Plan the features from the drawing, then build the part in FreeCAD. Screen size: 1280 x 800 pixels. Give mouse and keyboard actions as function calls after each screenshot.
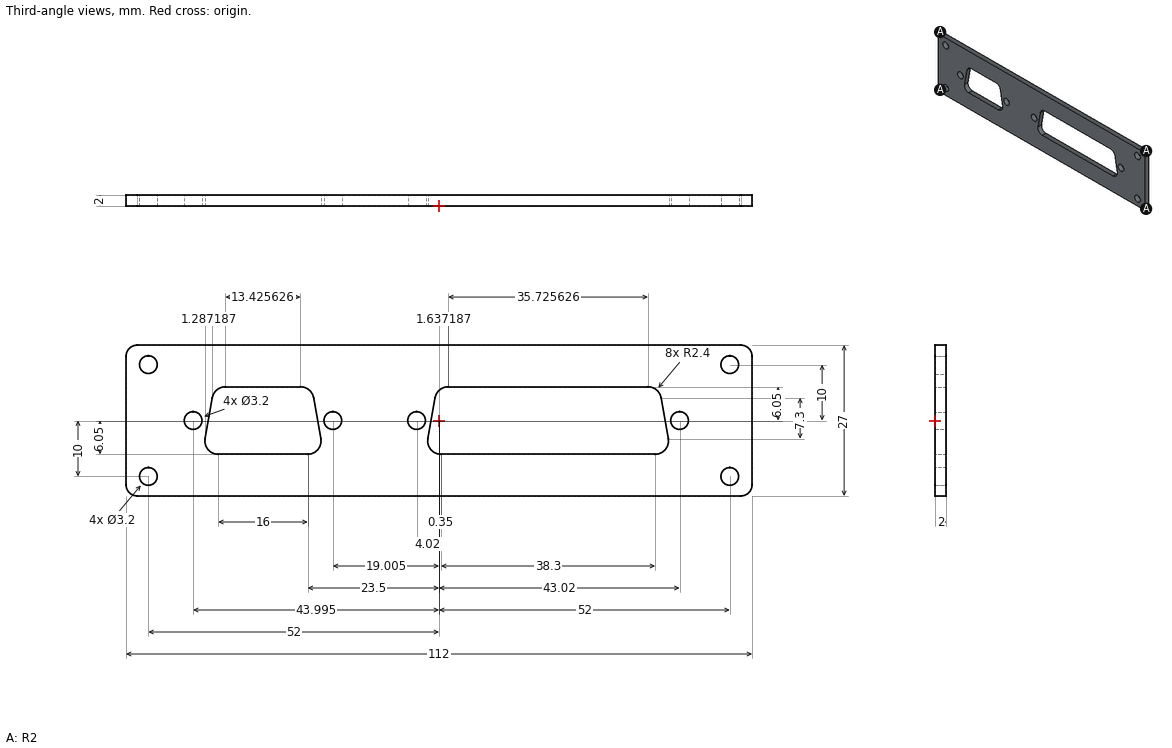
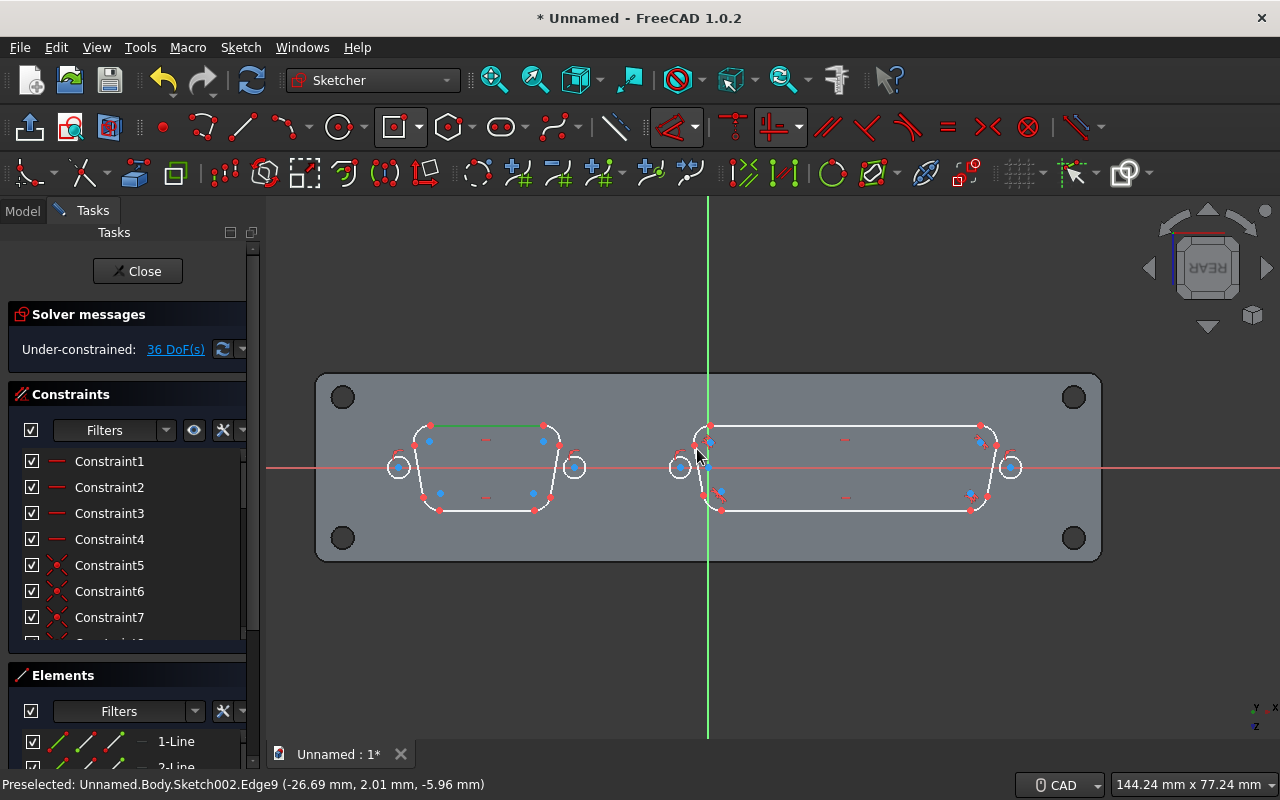
scroll(422, 428, up, 3)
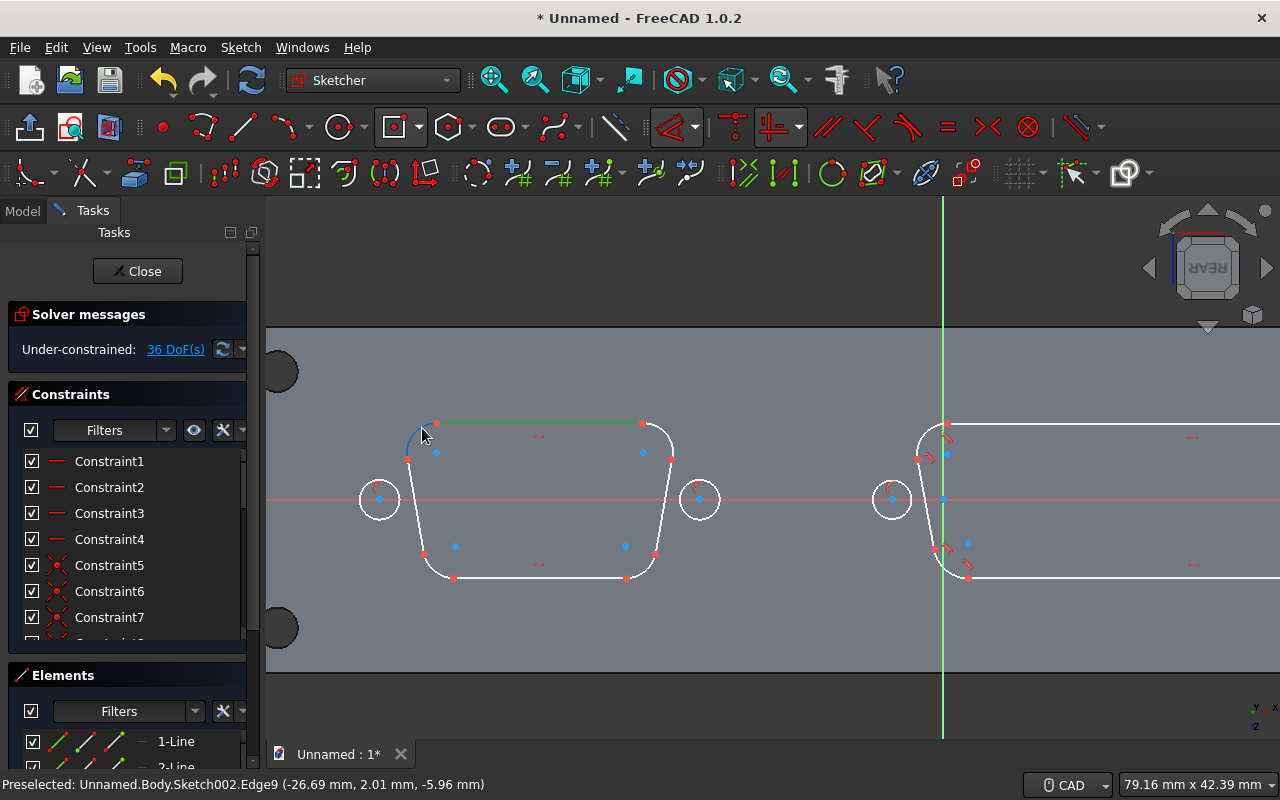
click(421, 427)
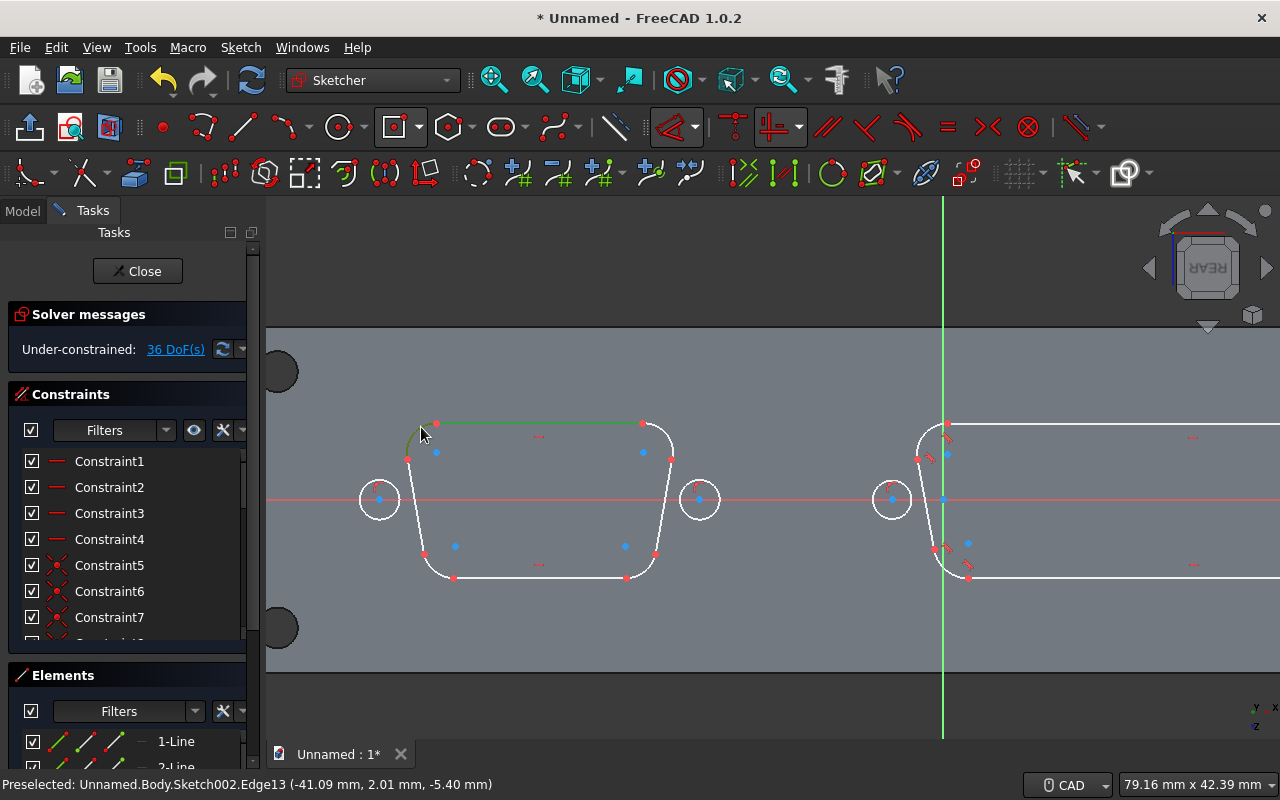
click(908, 128)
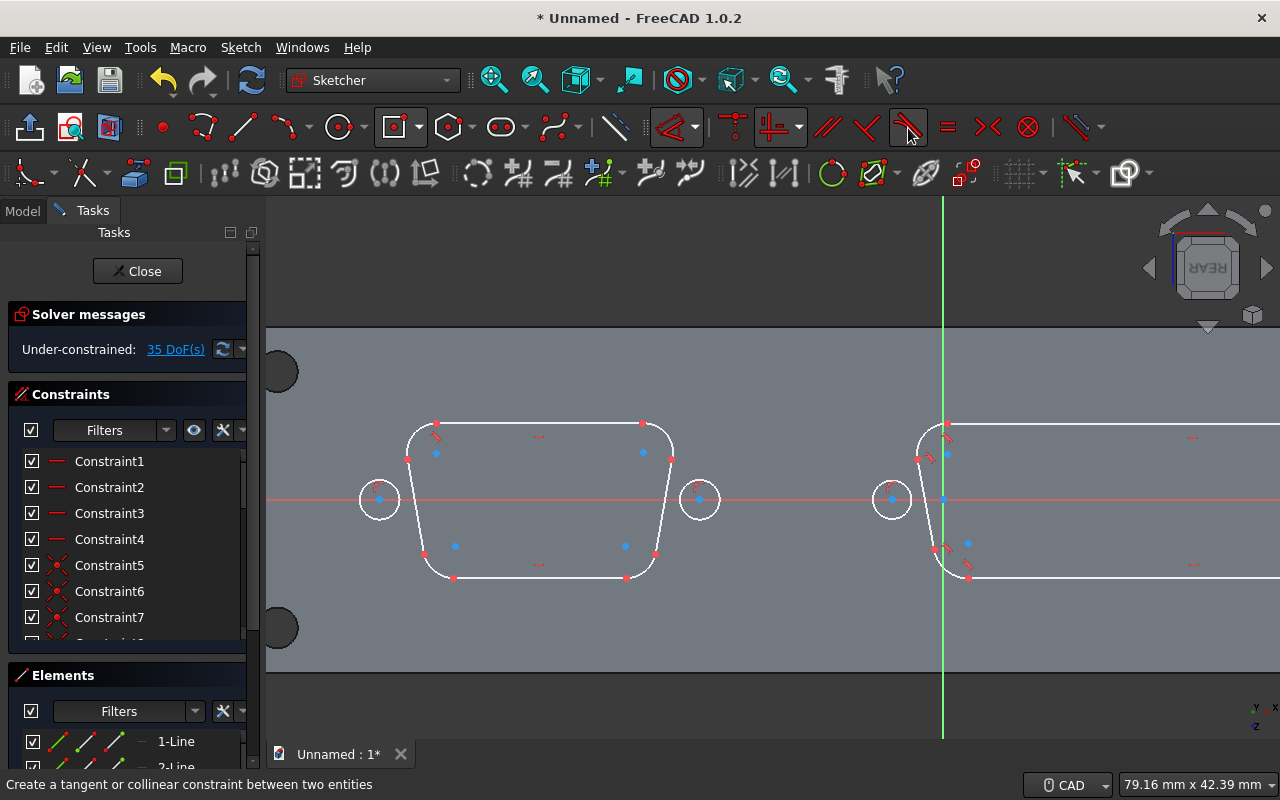
click(581, 423)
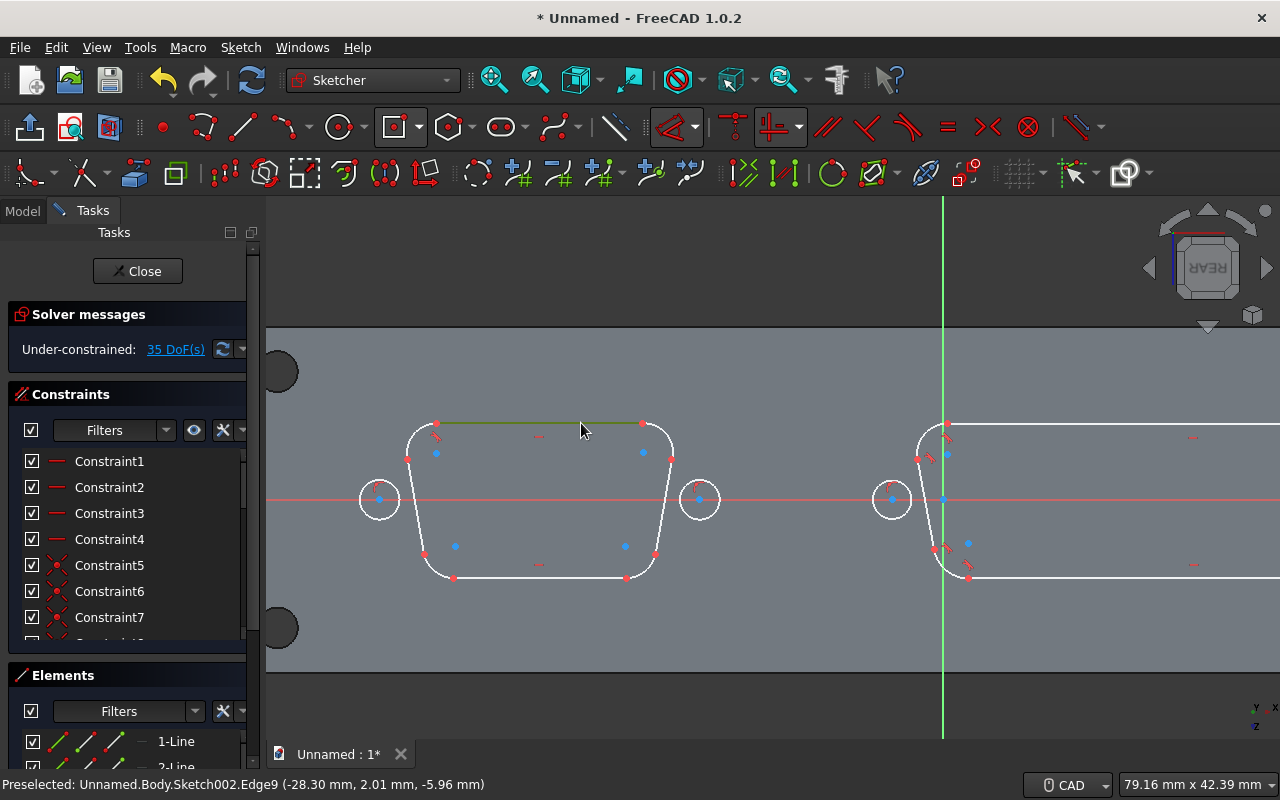
click(672, 444)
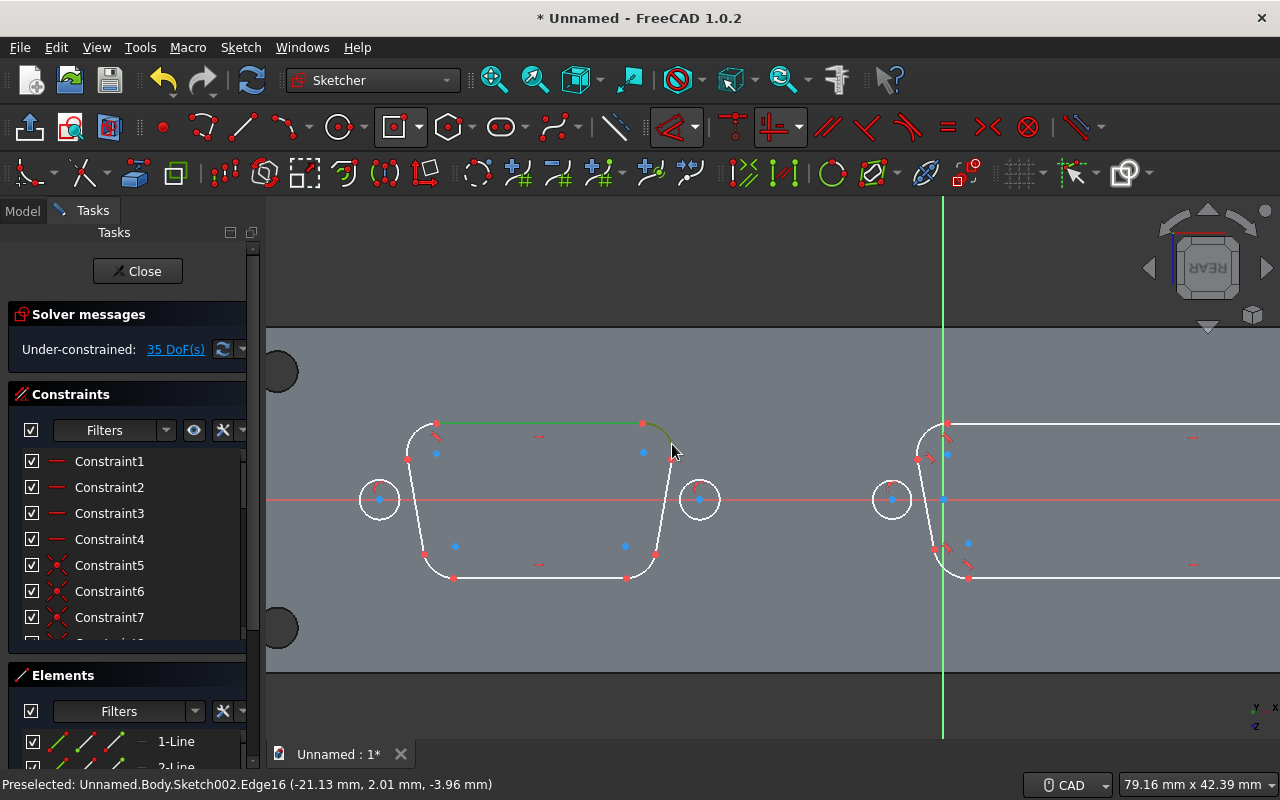
click(908, 128)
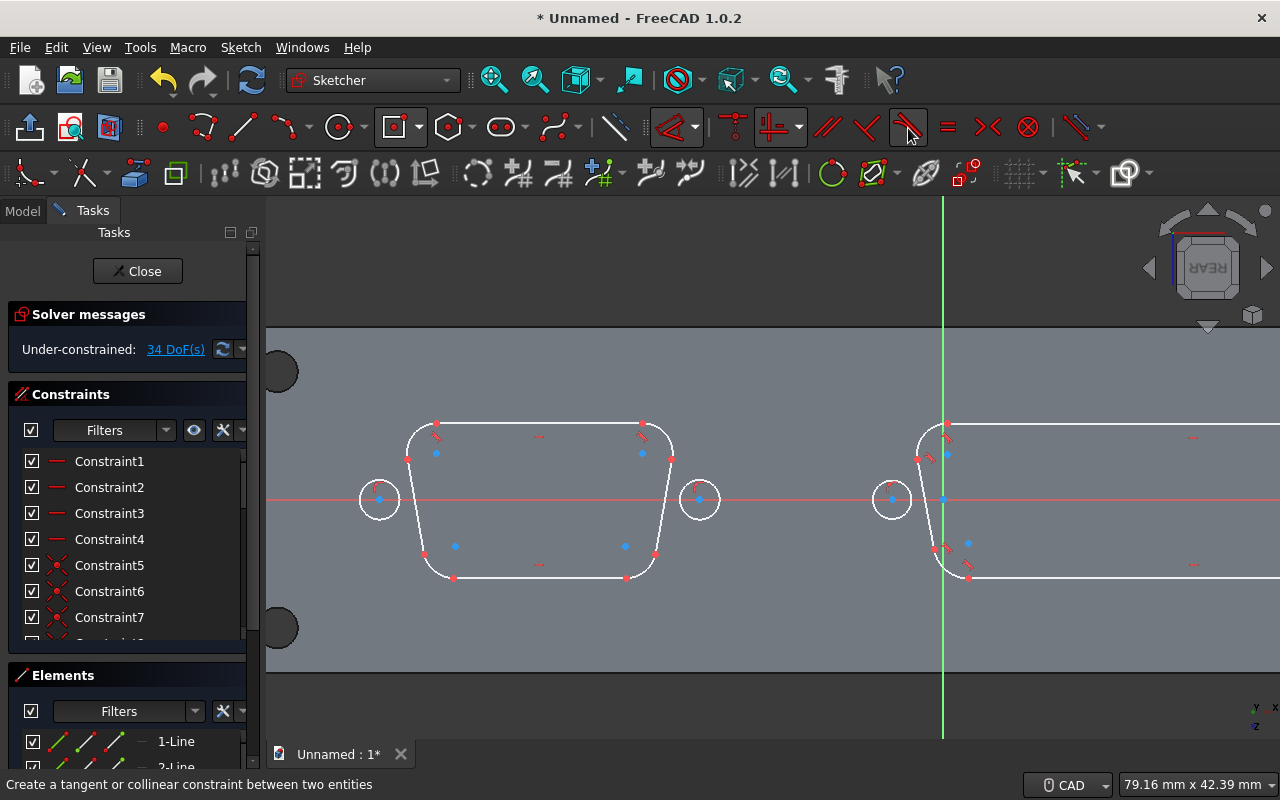
click(413, 488)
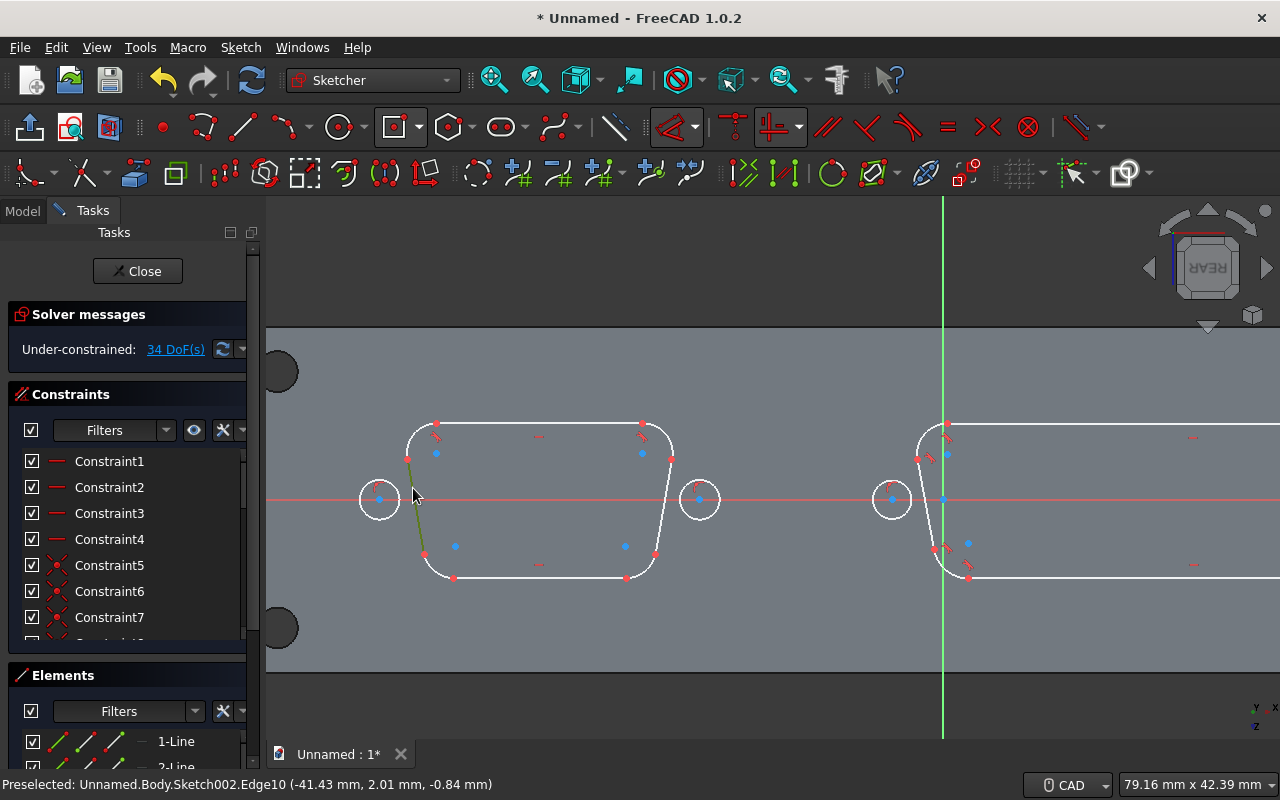
click(422, 428)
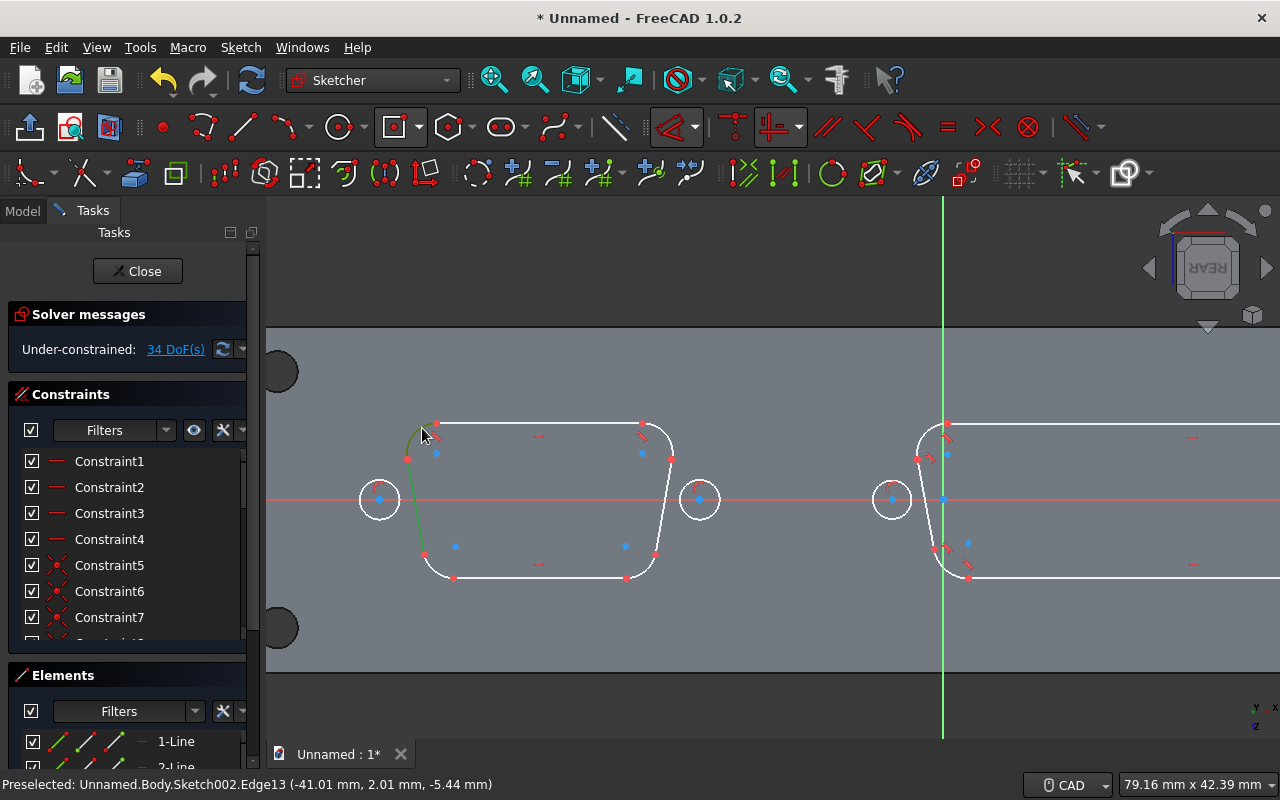
click(908, 128)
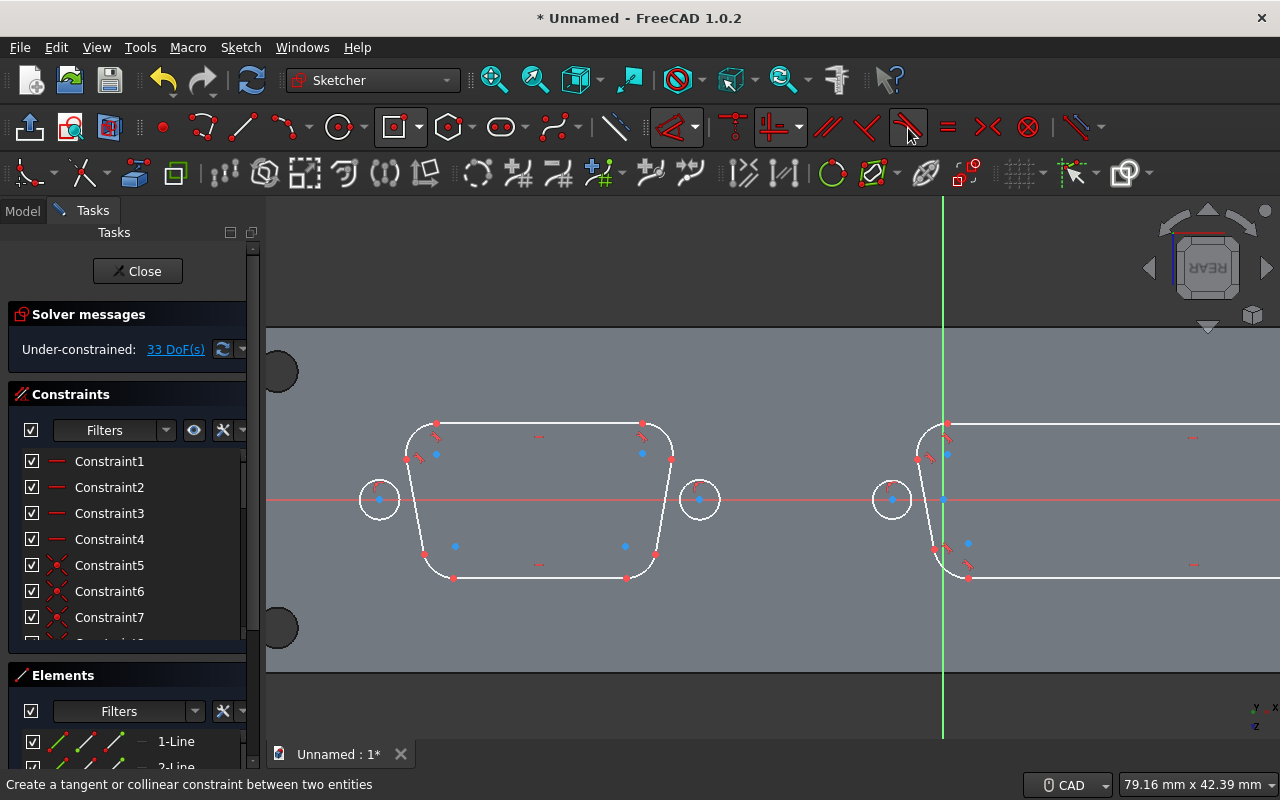
click(412, 488)